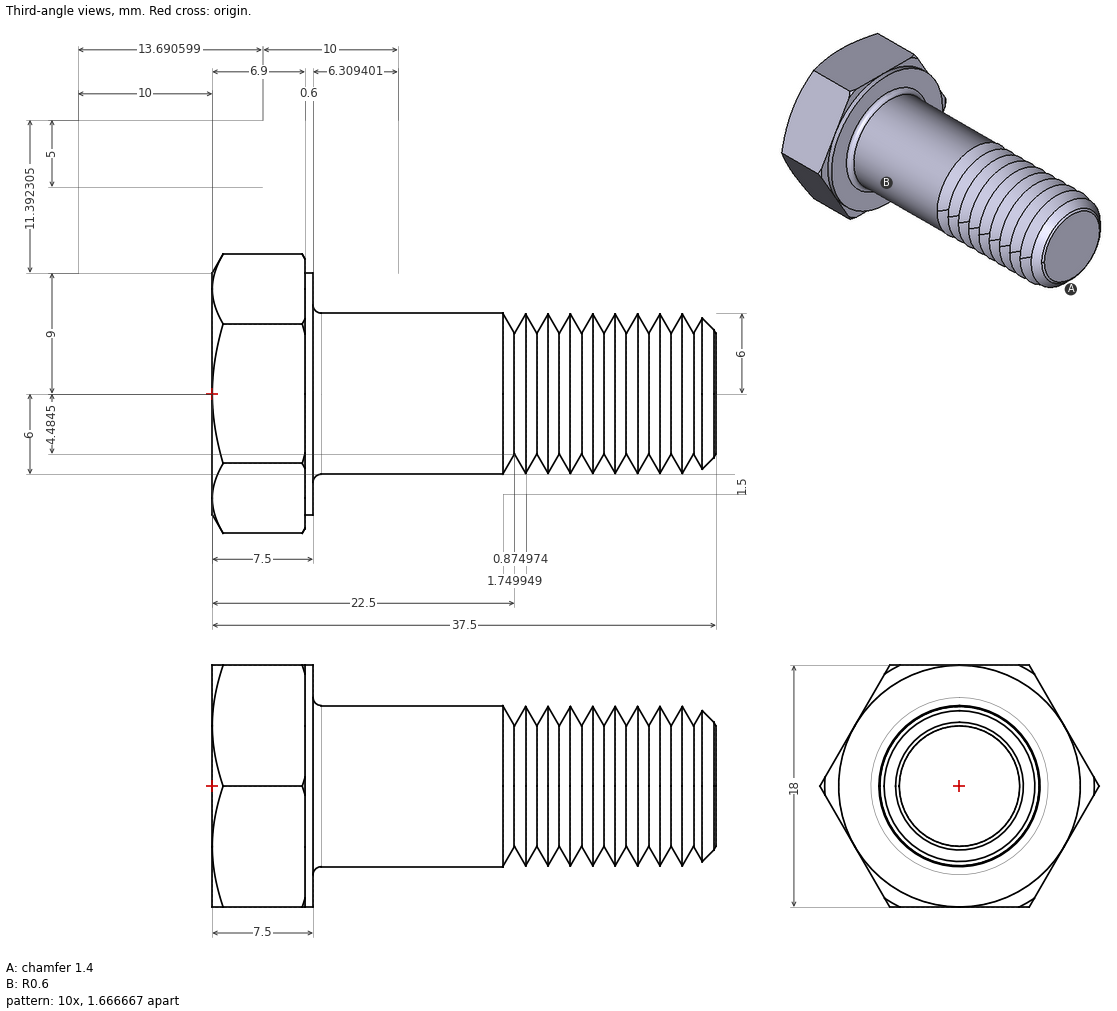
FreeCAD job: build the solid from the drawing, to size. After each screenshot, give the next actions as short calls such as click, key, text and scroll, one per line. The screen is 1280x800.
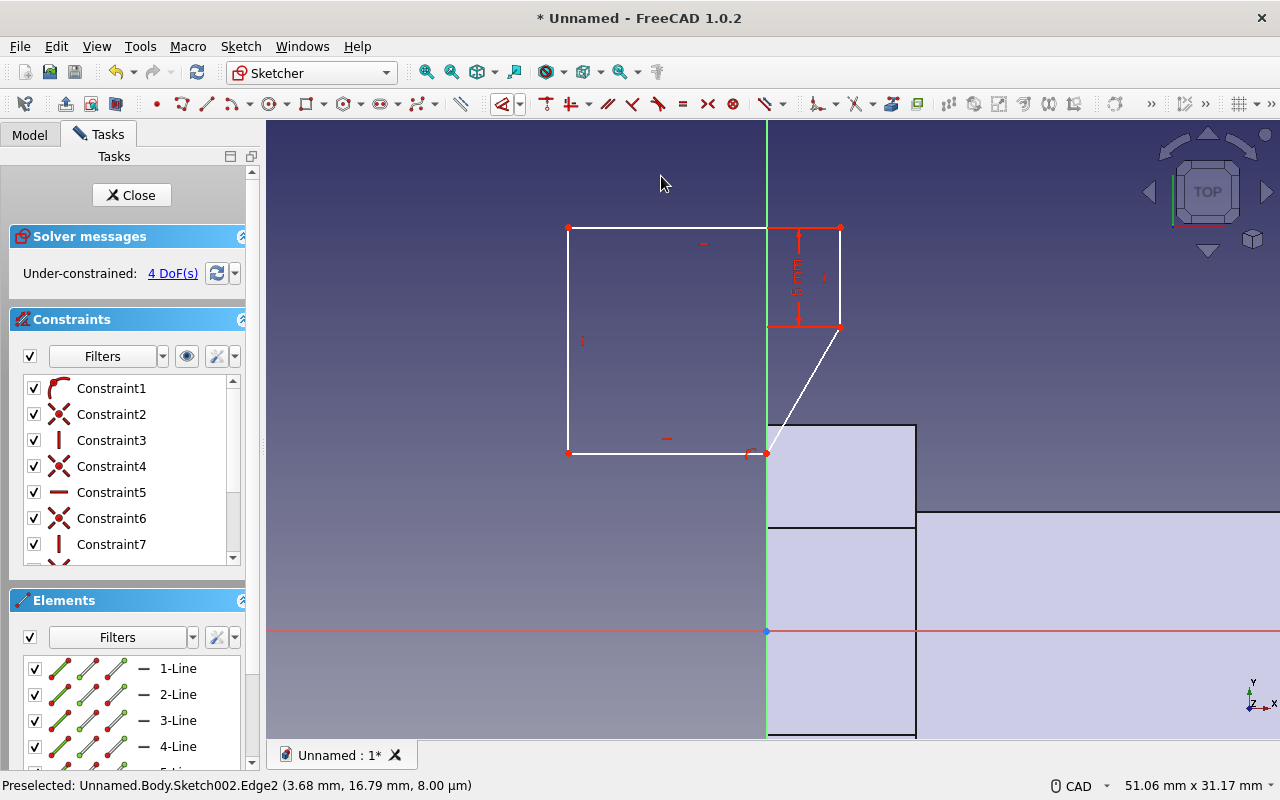
click(628, 454)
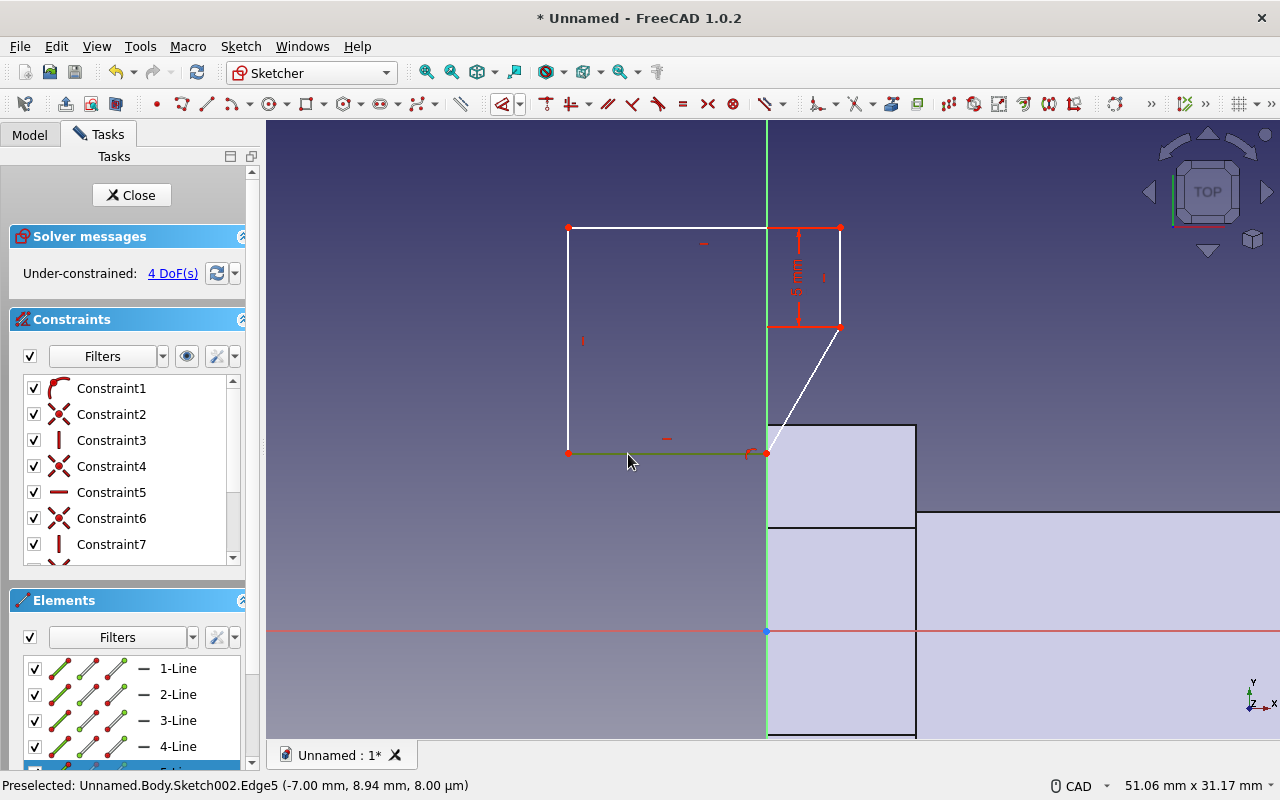
click(520, 104)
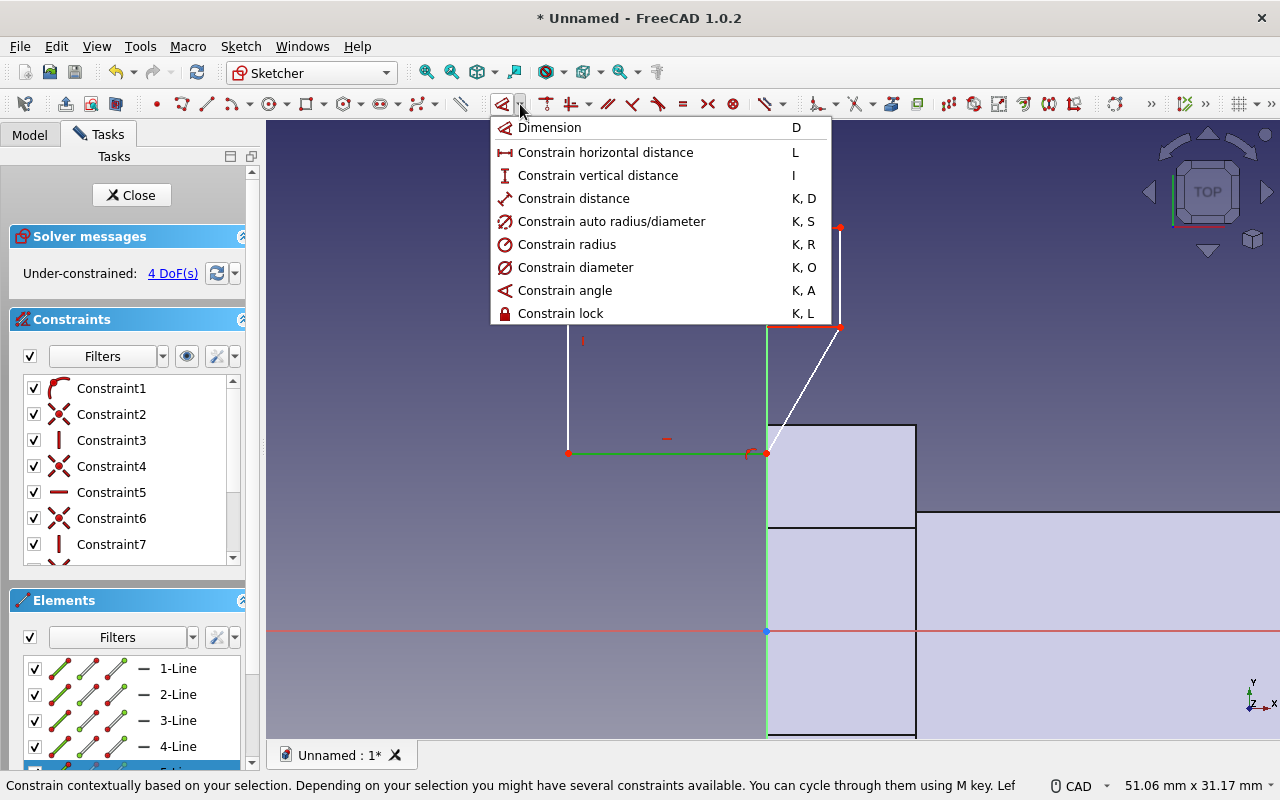
click(661, 152)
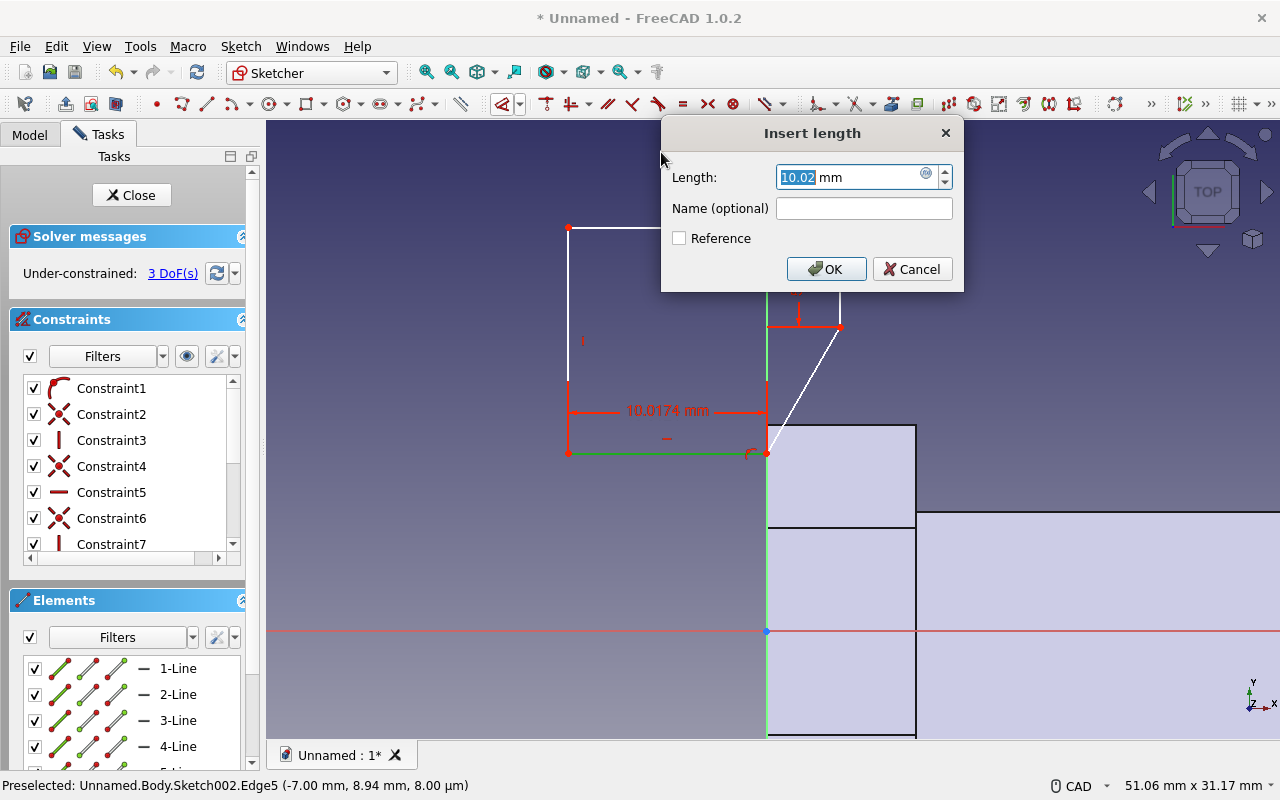
text(10)
key(Return)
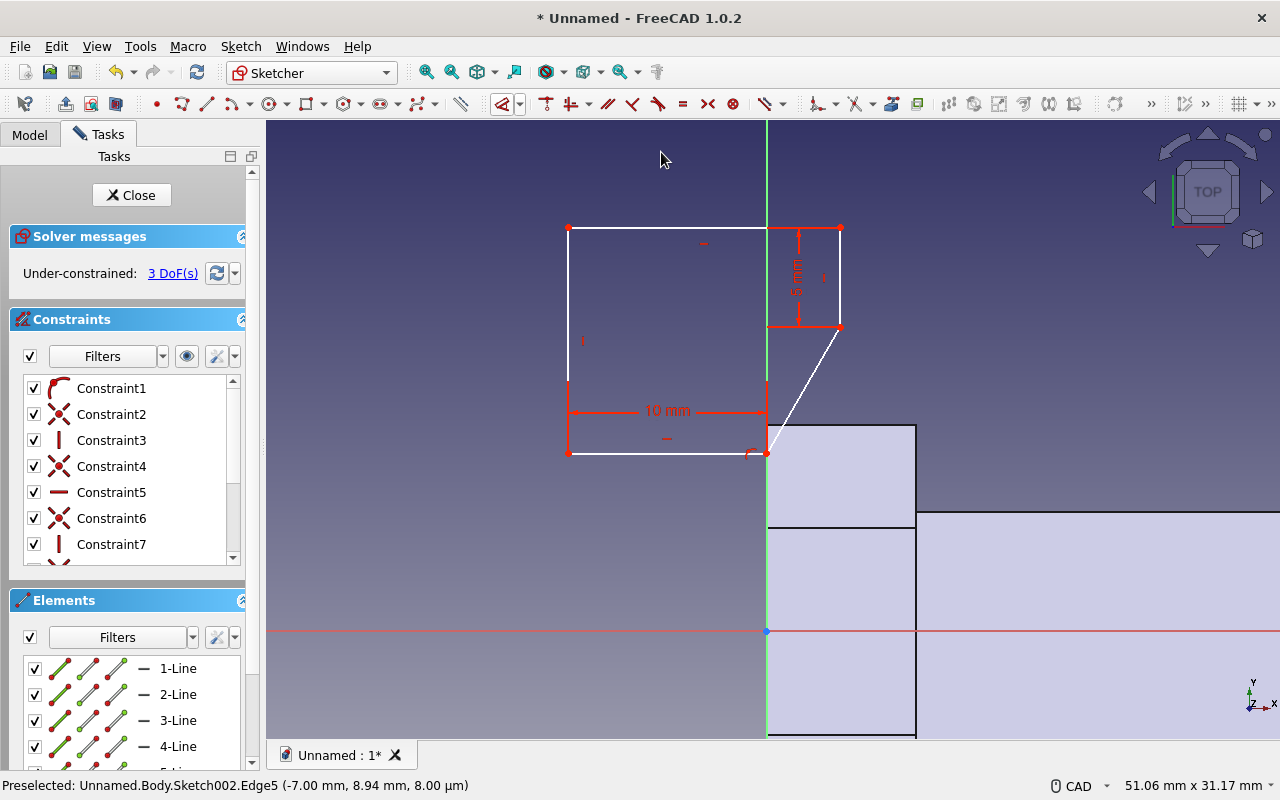
click(767, 454)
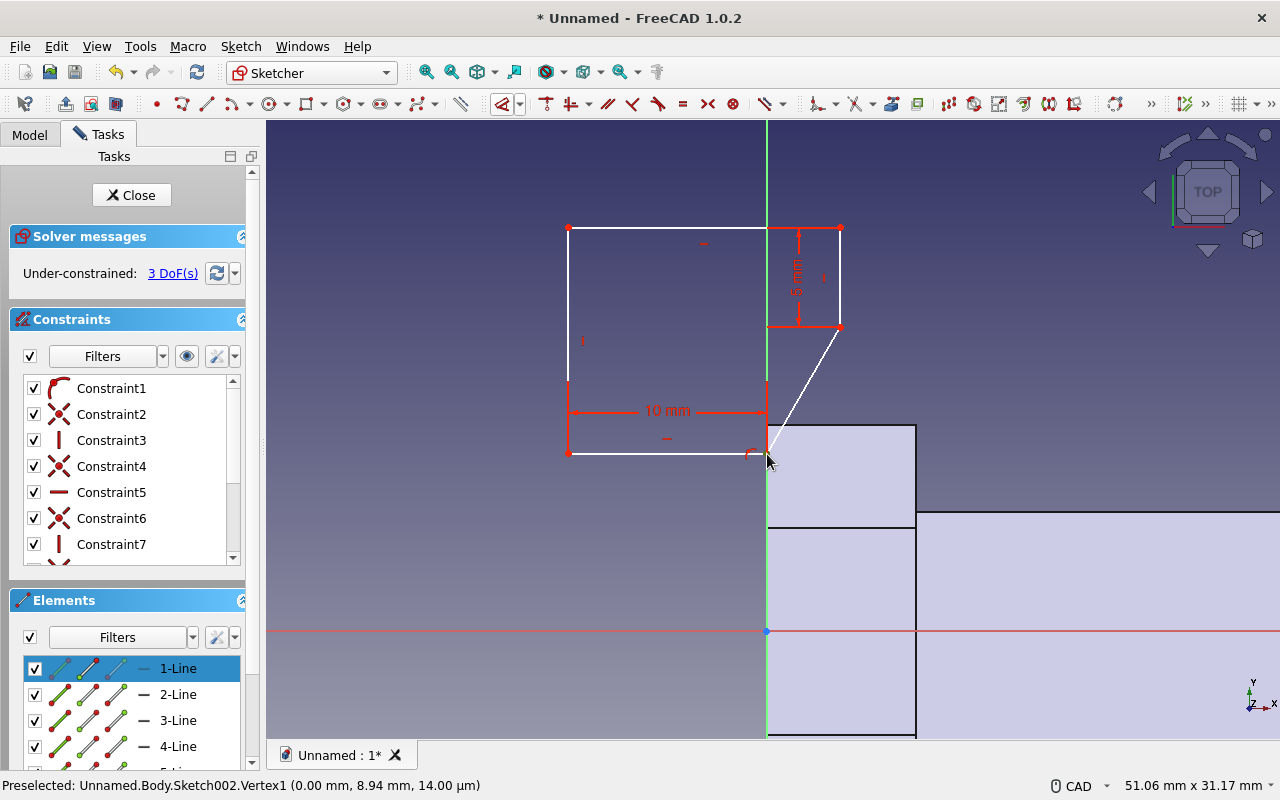
key(i)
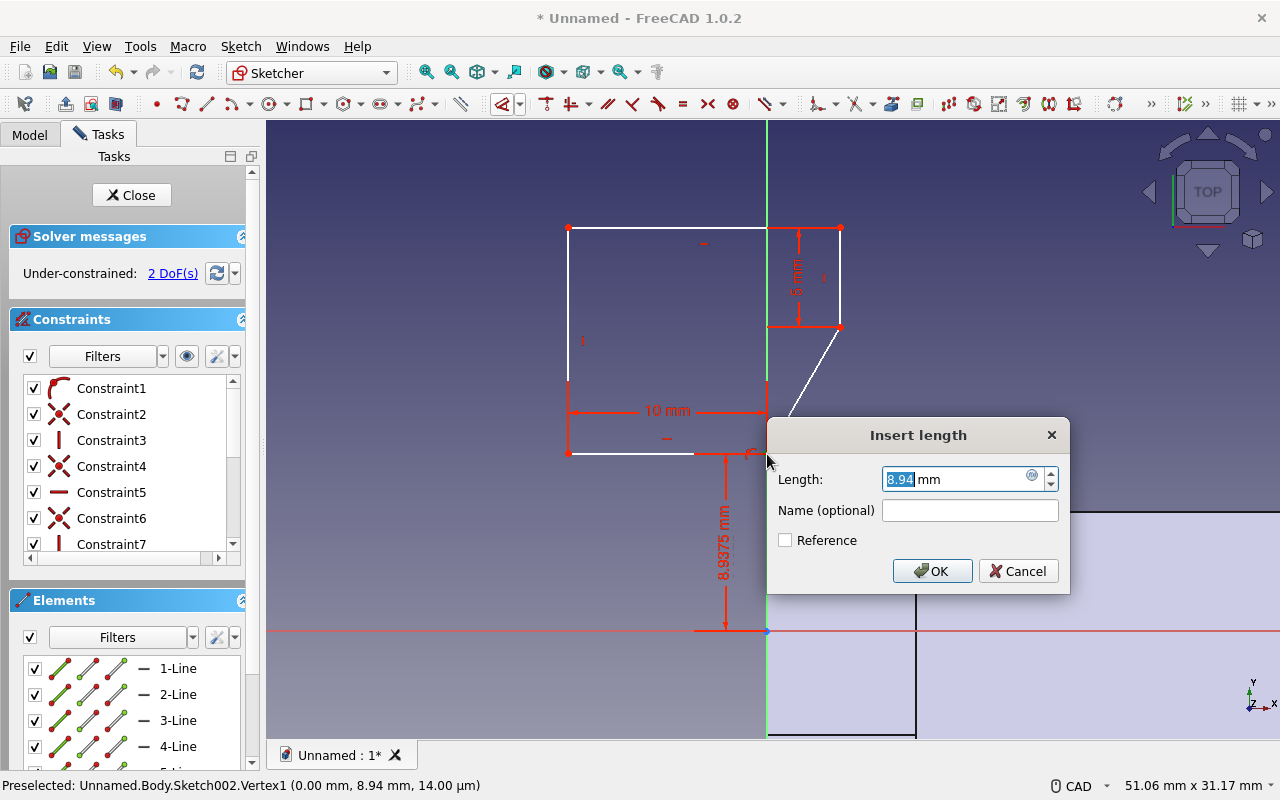
text(9)
key(Return)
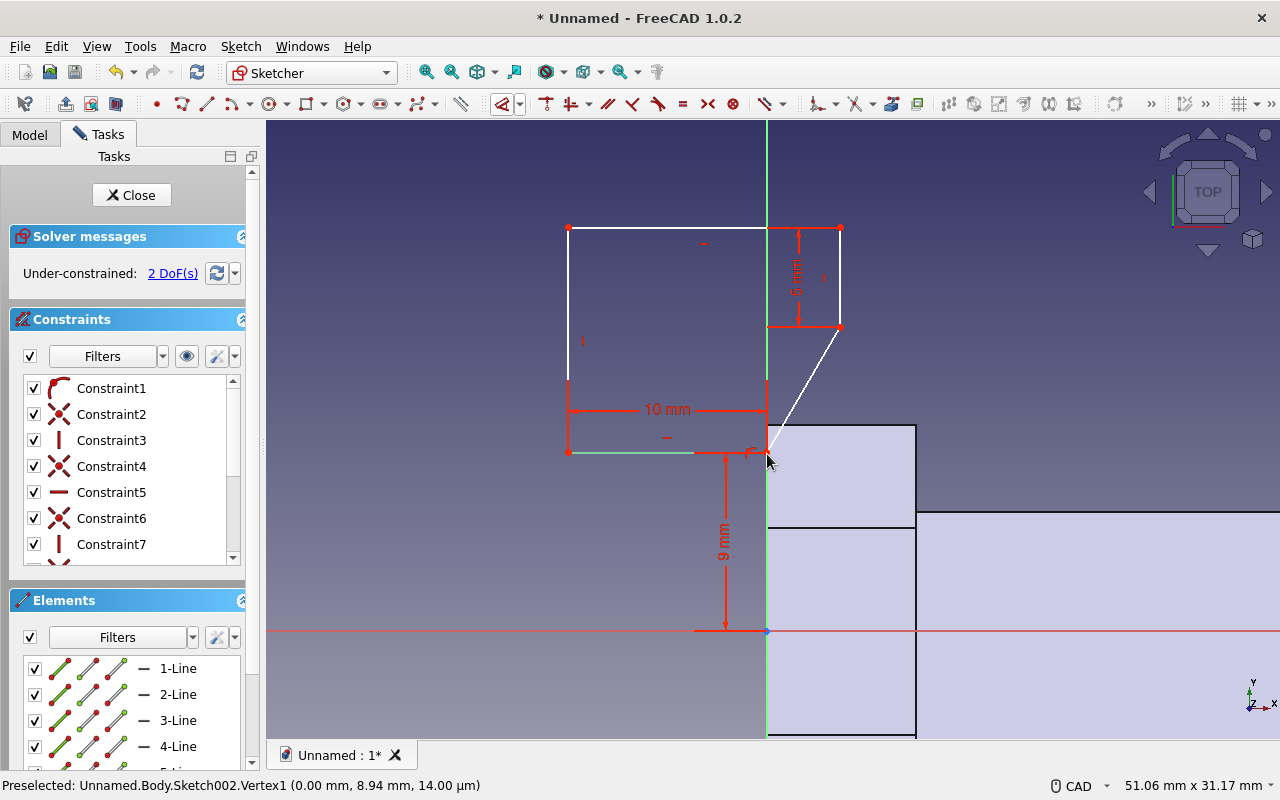
click(650, 228)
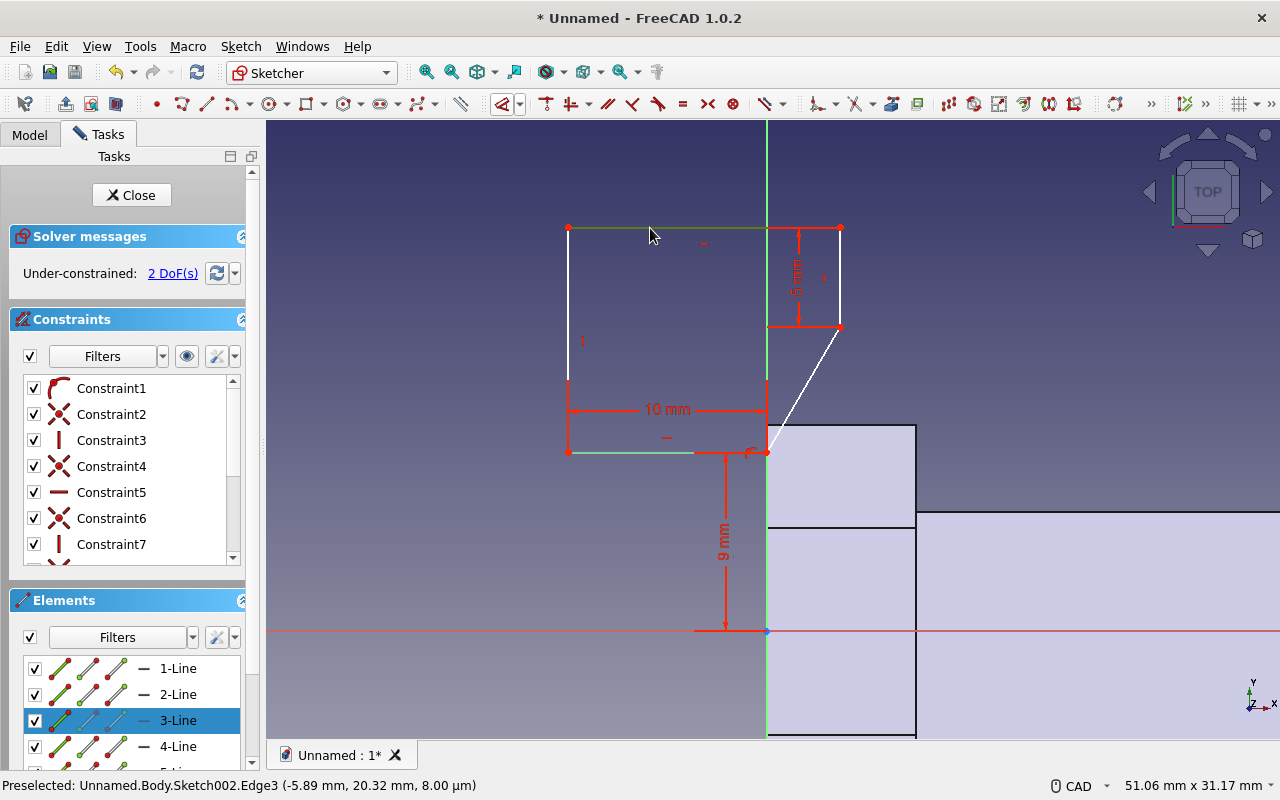
click(520, 104)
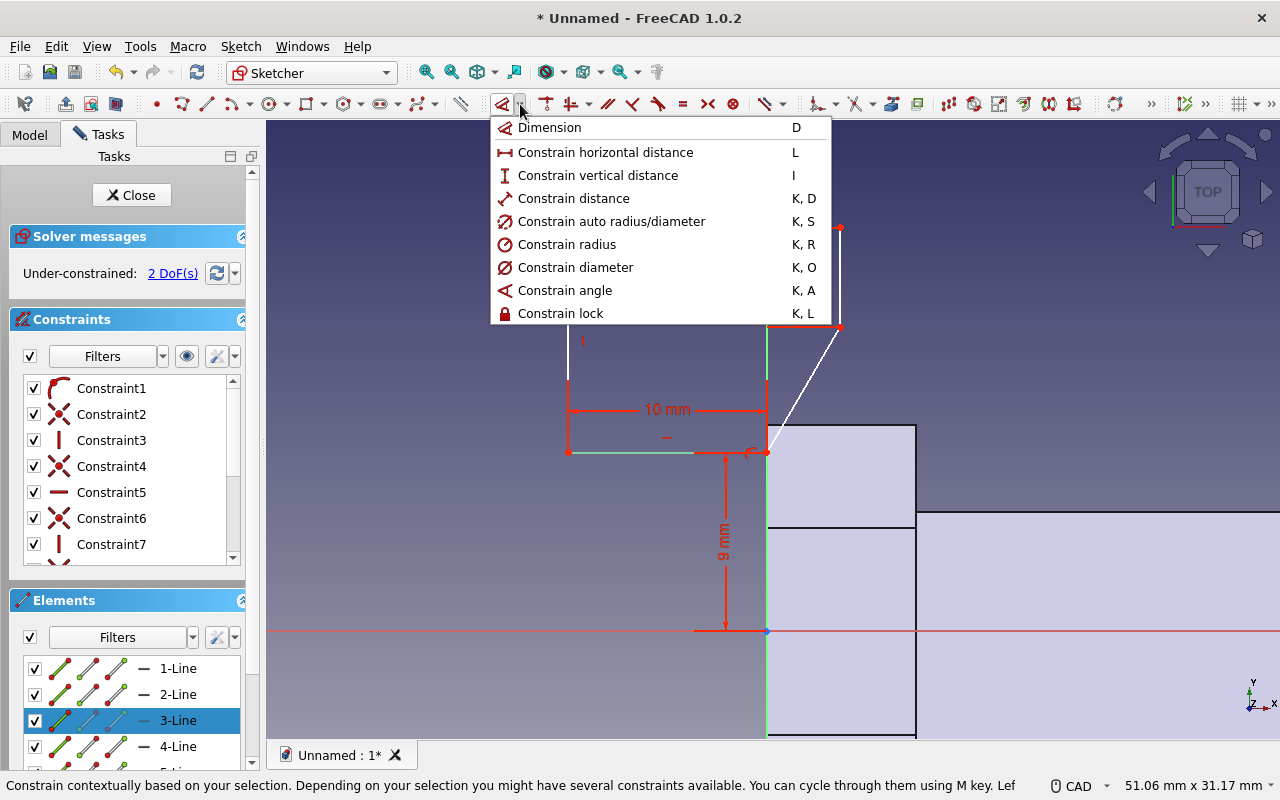
click(661, 152)